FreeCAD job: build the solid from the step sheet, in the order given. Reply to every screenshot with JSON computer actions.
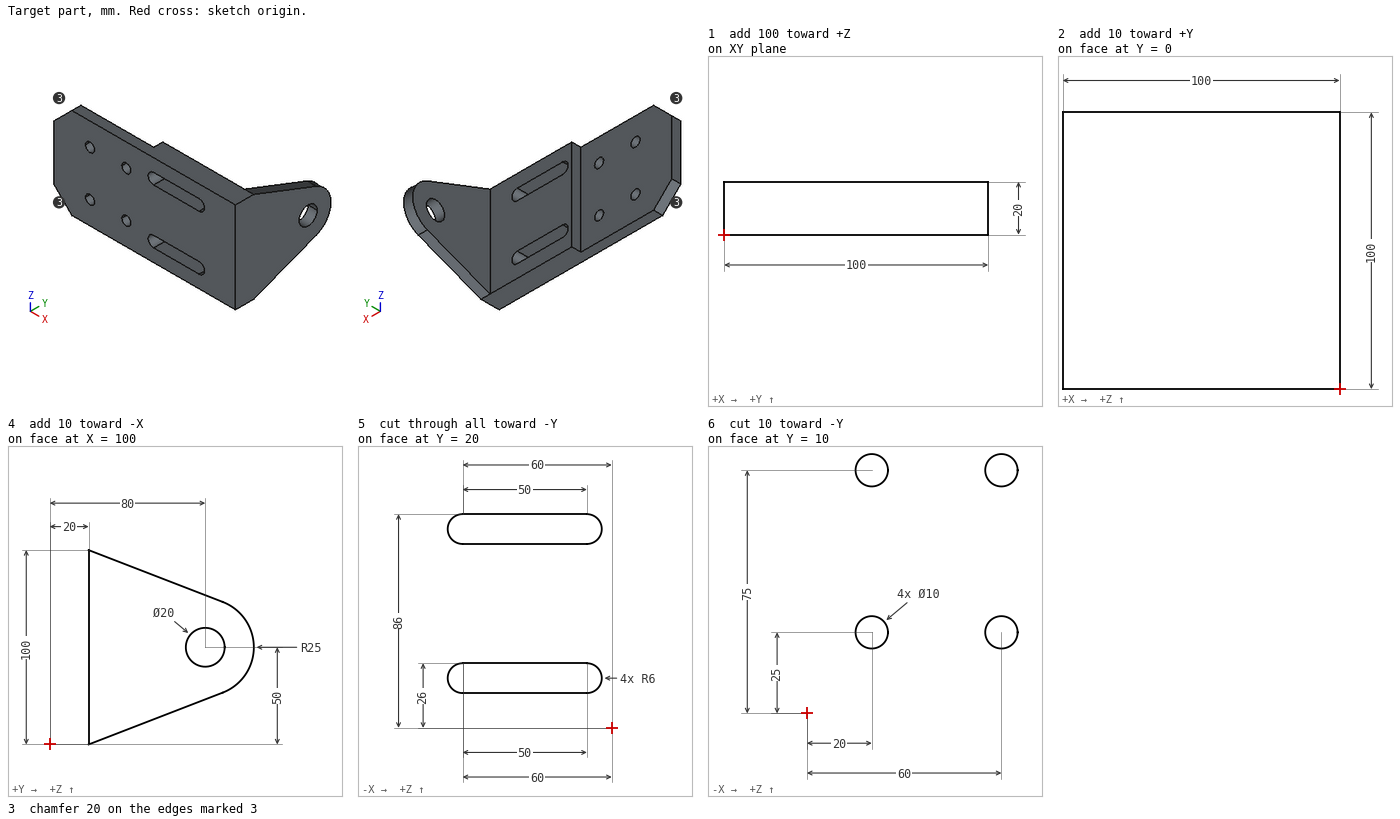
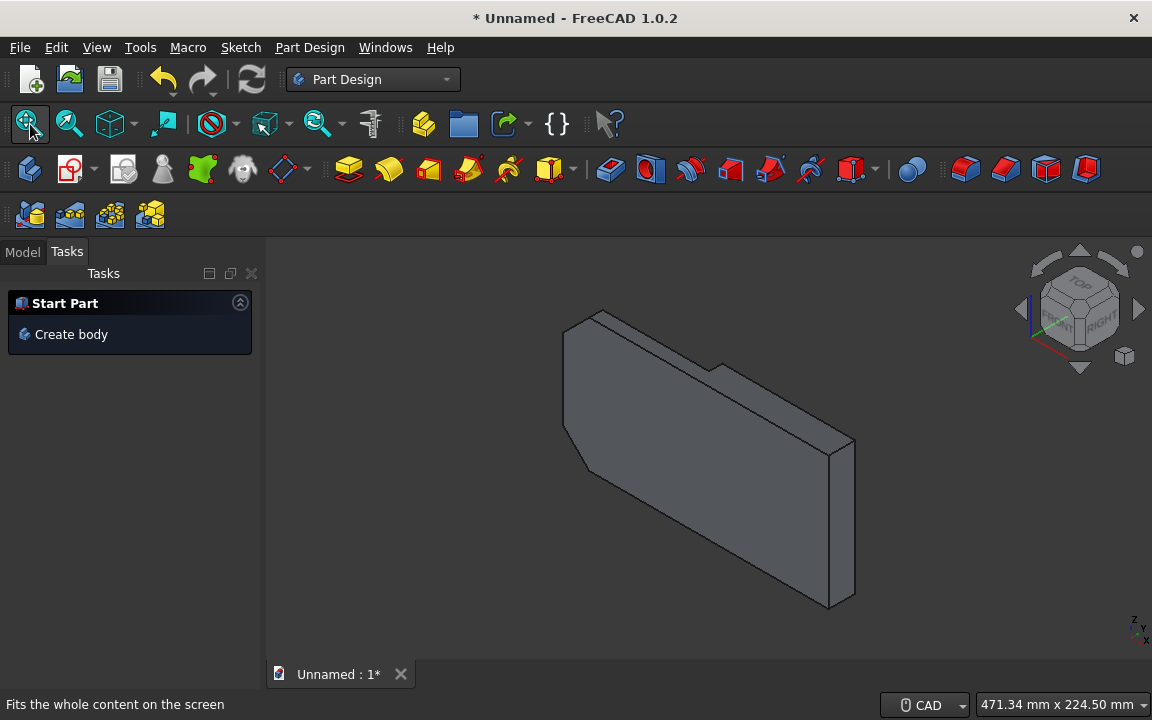
{"action": "left_click", "coordinate": [842, 480]}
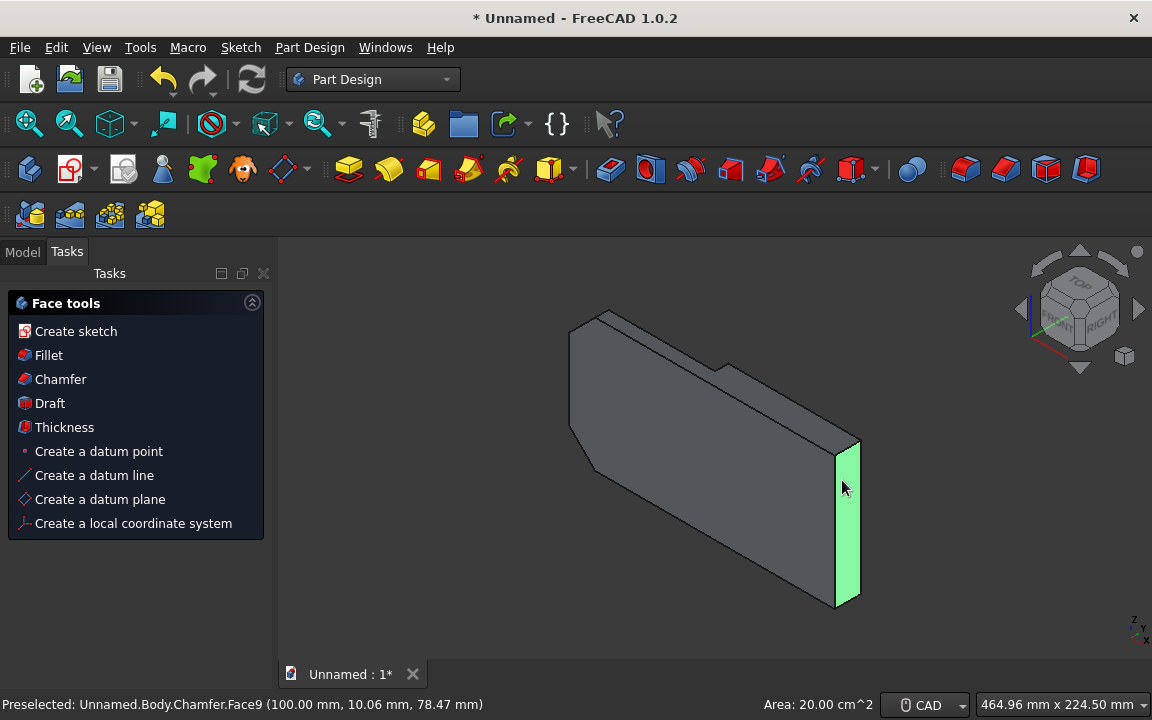
{"action": "left_click", "coordinate": [70, 170]}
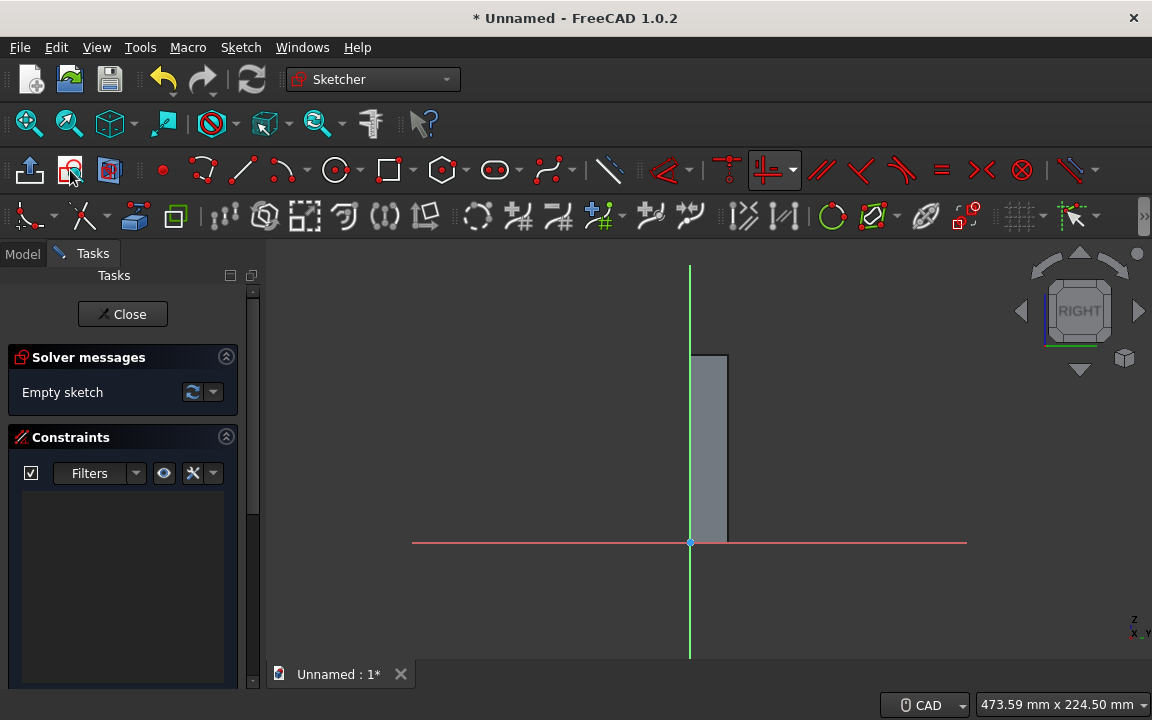
{"action": "scroll", "coordinate": [987, 449], "scroll_direction": "up", "scroll_amount": 2}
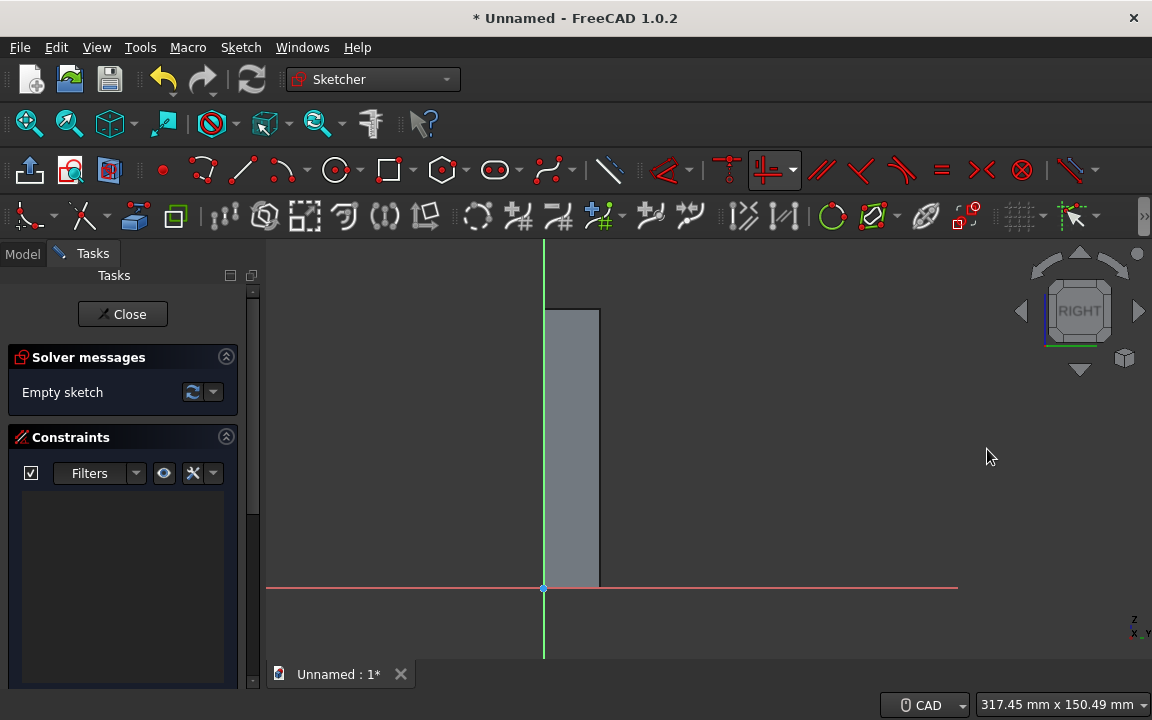
{"action": "left_click", "coordinate": [204, 170]}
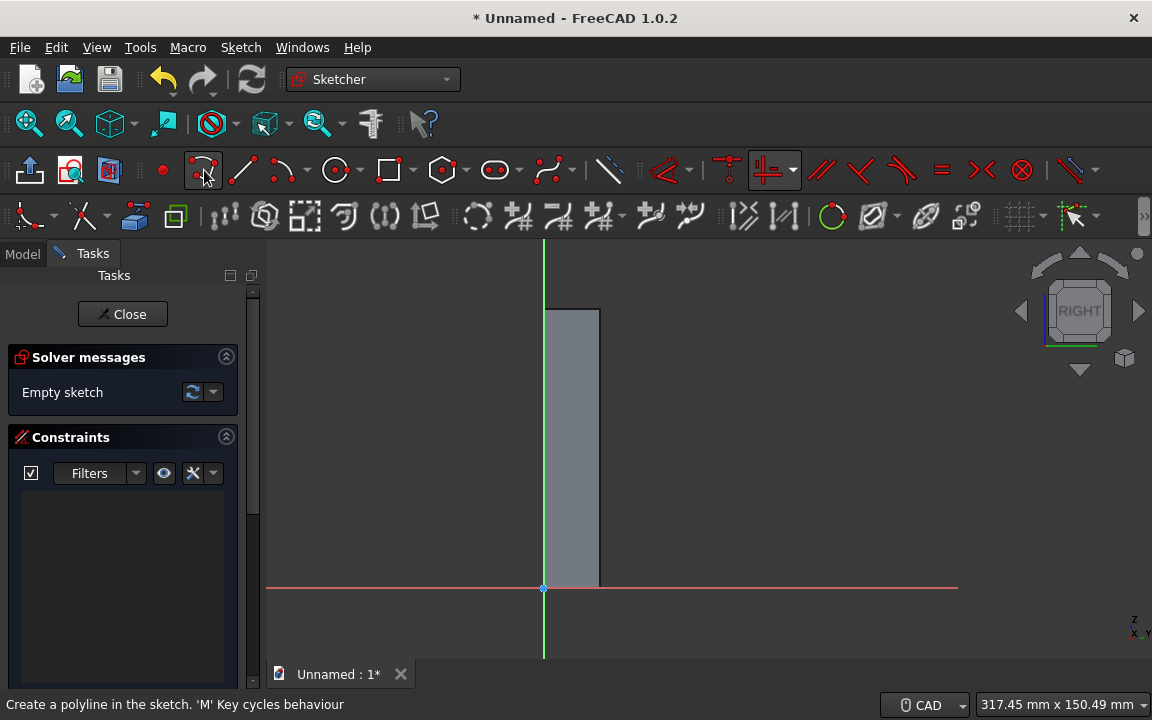
{"action": "left_click", "coordinate": [792, 384]}
{"action": "left_click", "coordinate": [600, 309]}
{"action": "left_click", "coordinate": [600, 588]}
{"action": "left_click", "coordinate": [792, 514]}
{"action": "right_click", "coordinate": [792, 514]}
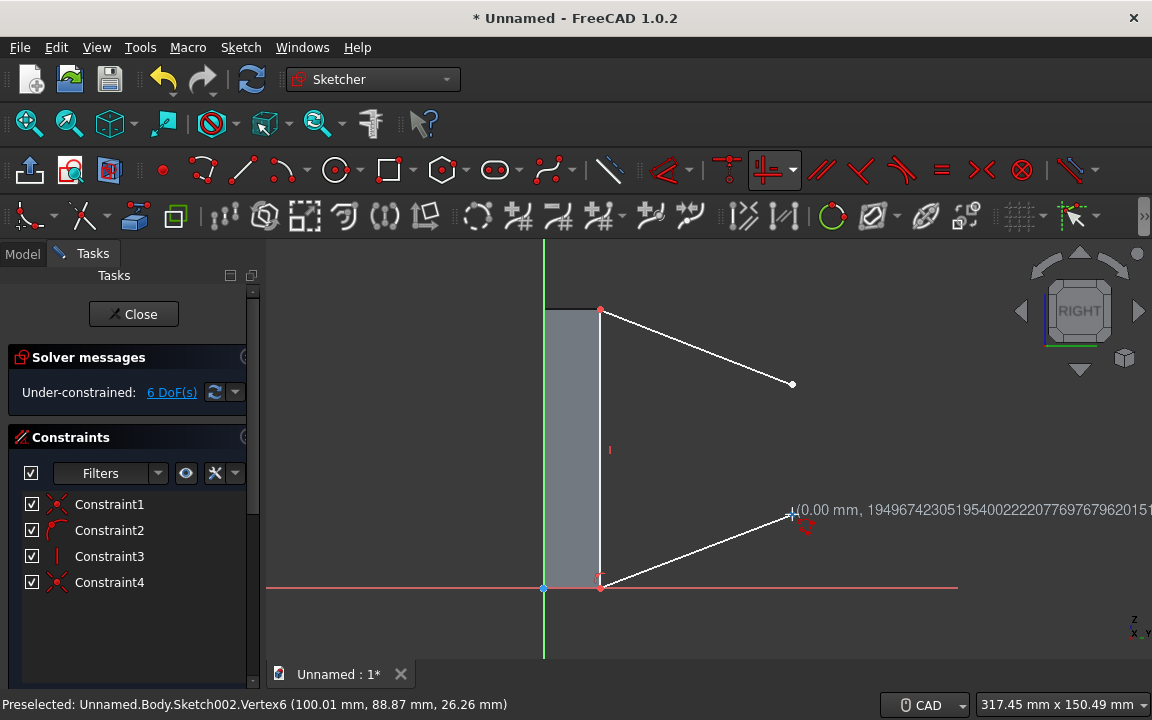
{"action": "left_click", "coordinate": [310, 170]}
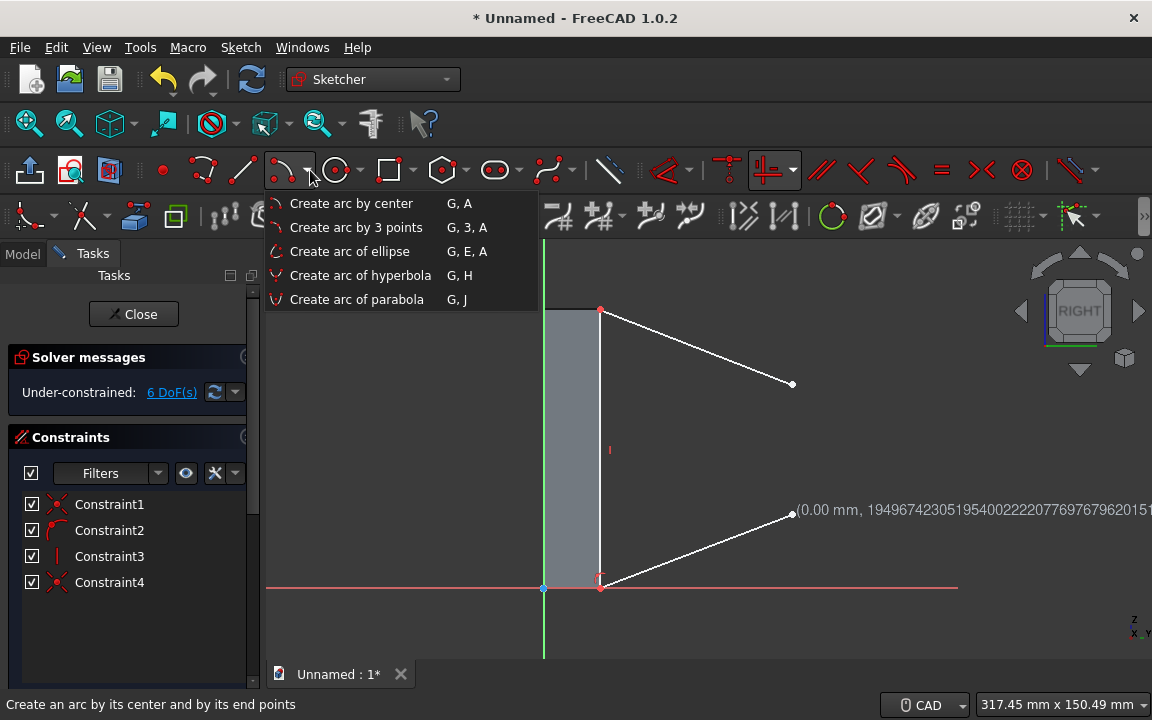
{"action": "left_click", "coordinate": [402, 227]}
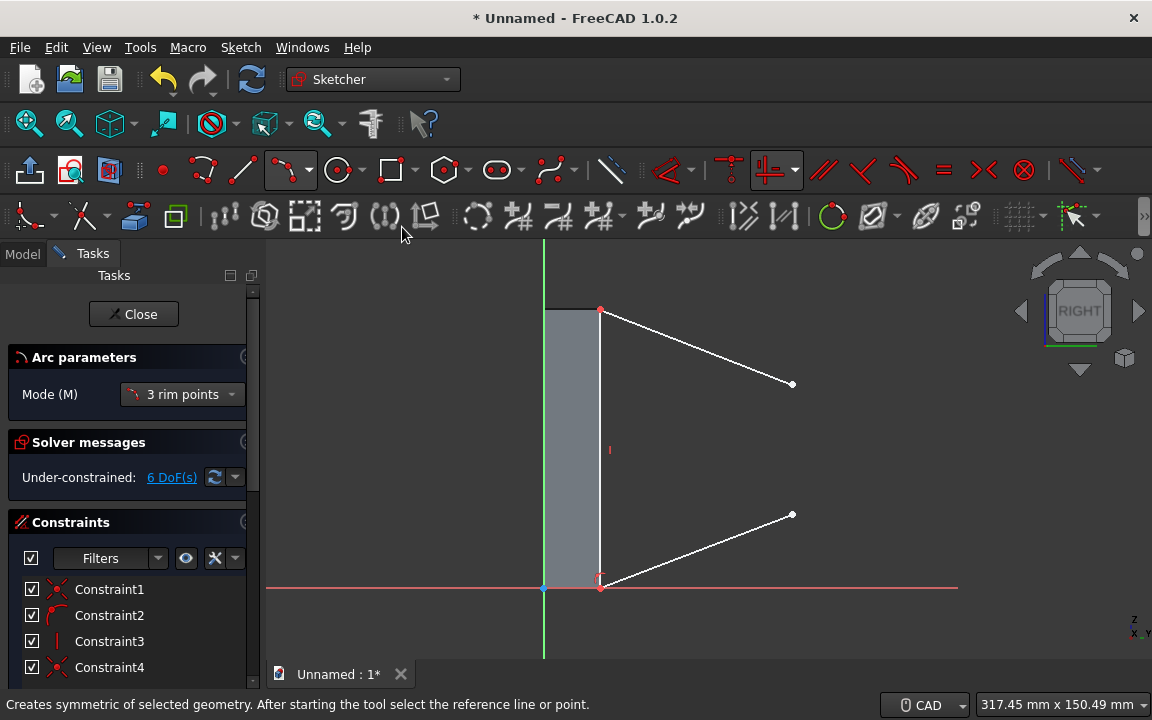
{"action": "left_click", "coordinate": [792, 515]}
{"action": "left_click", "coordinate": [792, 385]}
{"action": "left_click", "coordinate": [837, 449]}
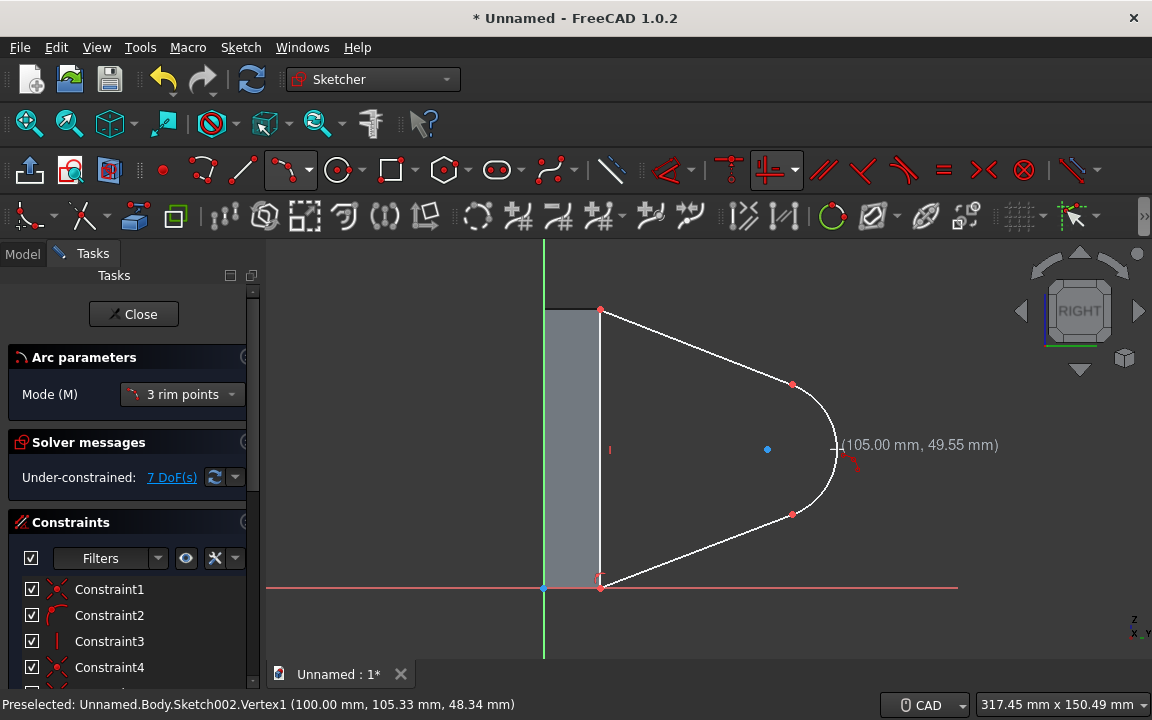
{"action": "left_click", "coordinate": [338, 170]}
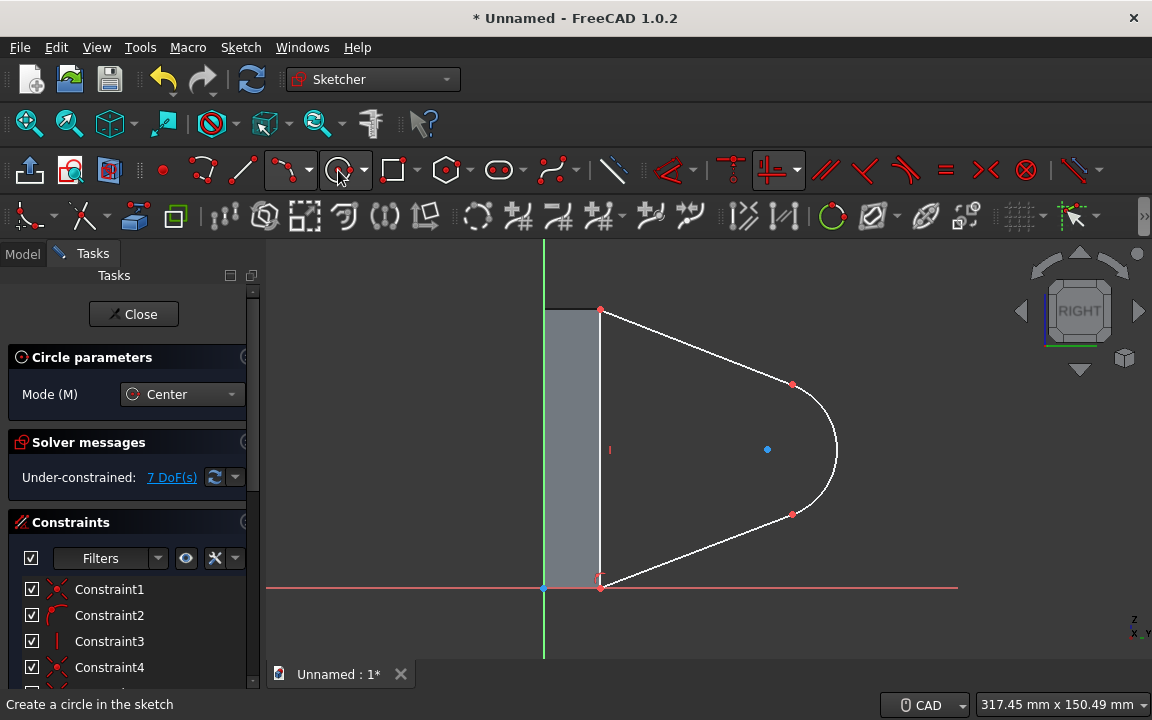
{"action": "left_click", "coordinate": [767, 449]}
{"action": "left_click", "coordinate": [787, 429]}
{"action": "key", "text": "Escape"}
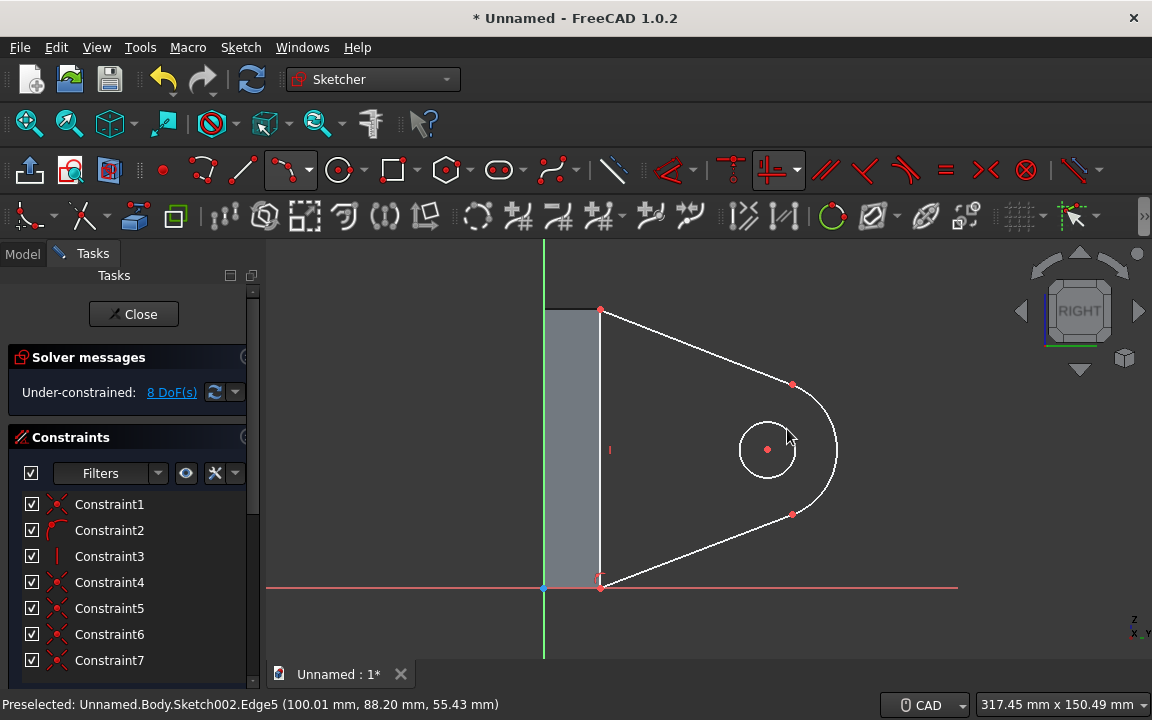
{"action": "left_click", "coordinate": [734, 363]}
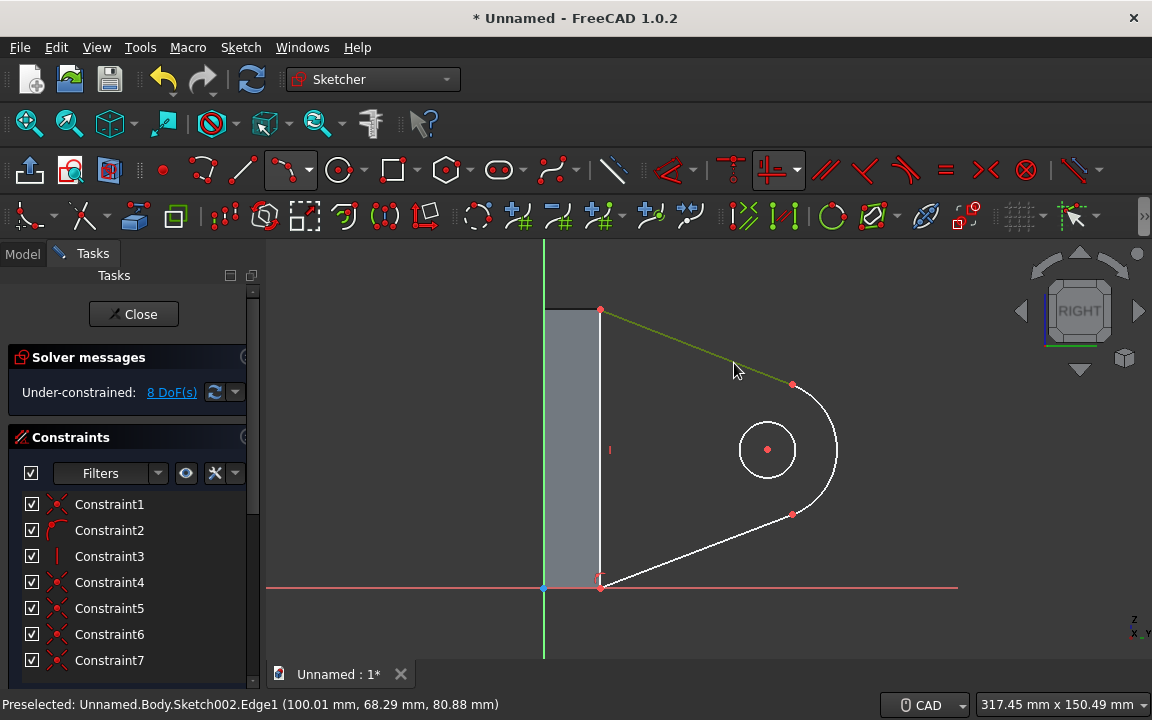
{"action": "left_click", "coordinate": [829, 482]}